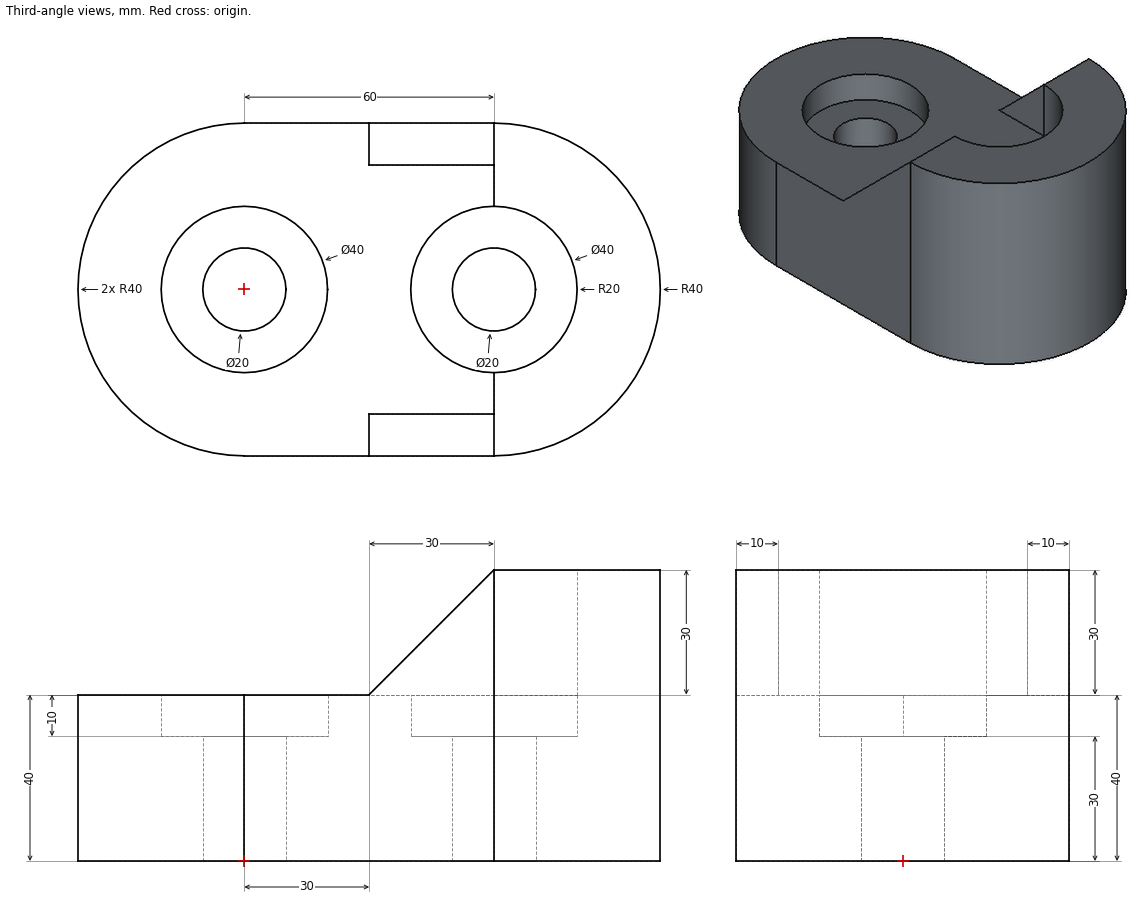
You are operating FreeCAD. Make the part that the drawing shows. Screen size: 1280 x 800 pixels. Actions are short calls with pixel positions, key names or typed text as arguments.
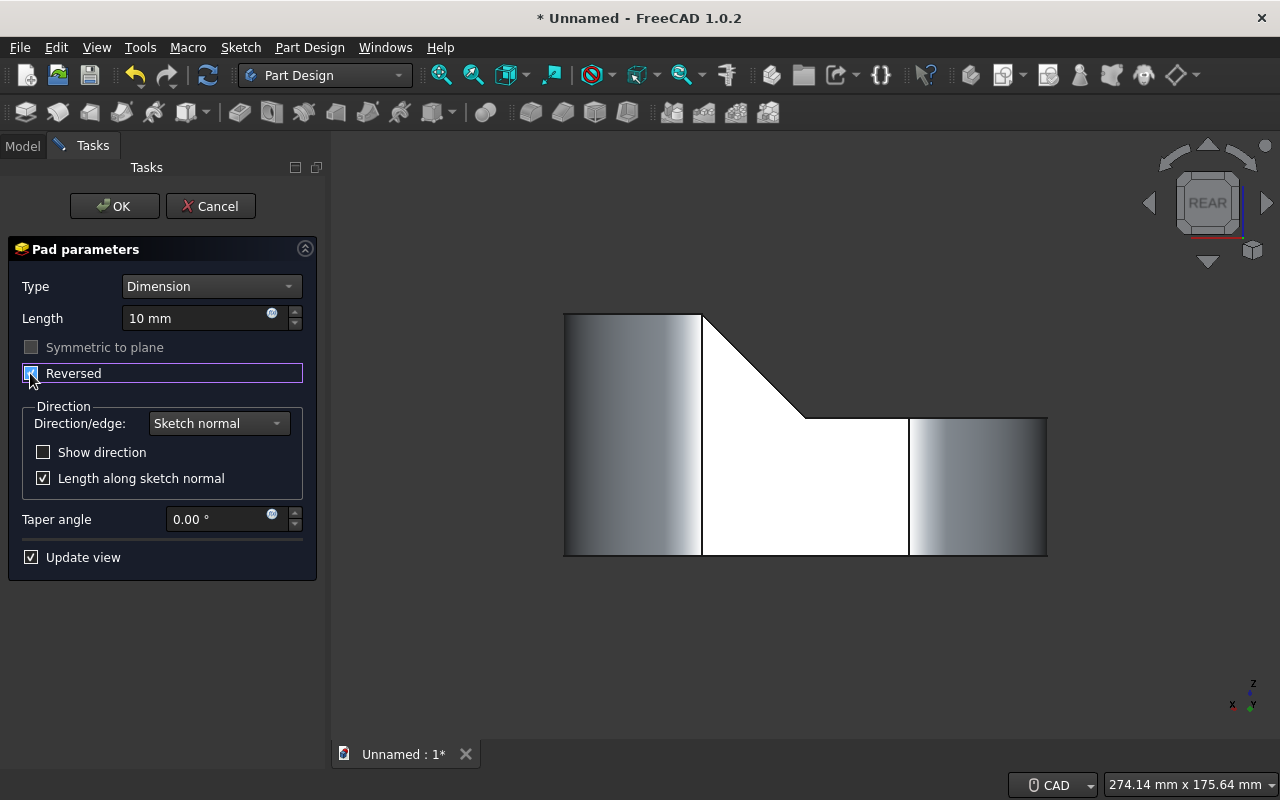
click(115, 206)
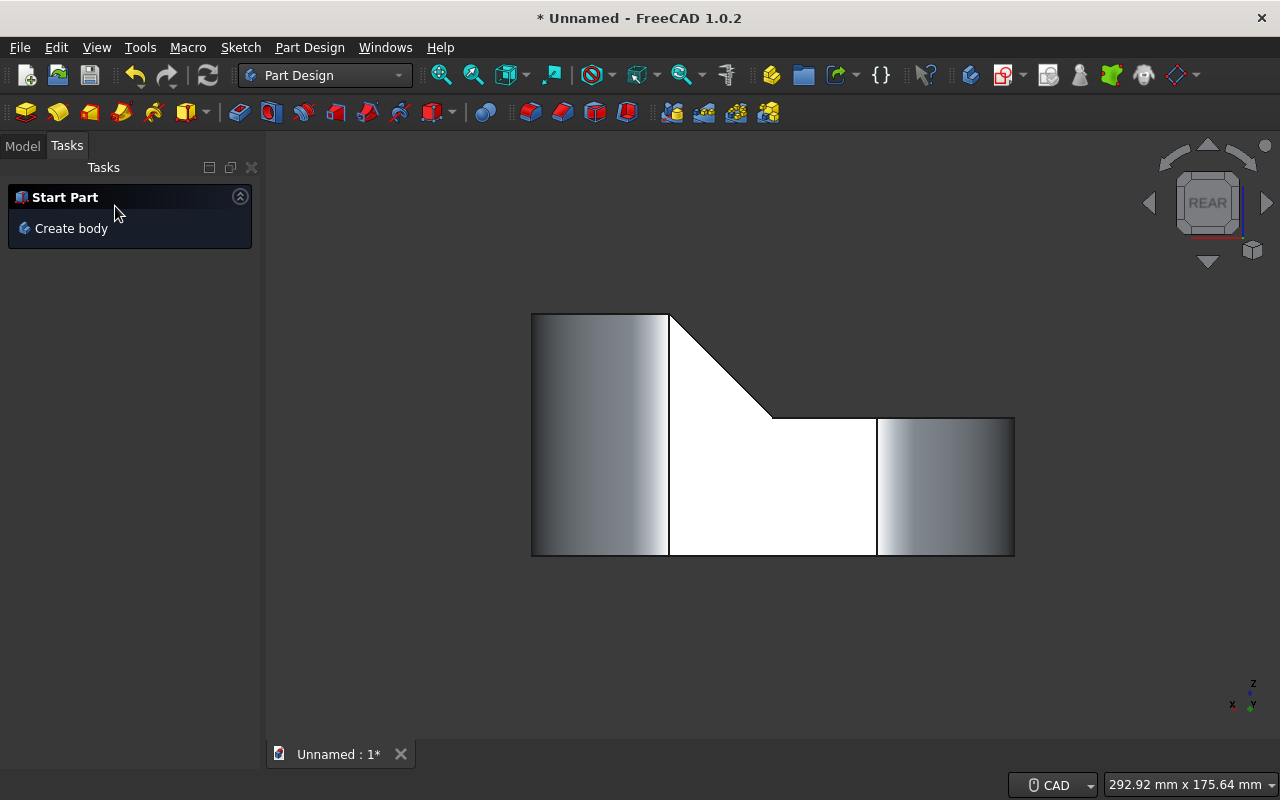
key(0)